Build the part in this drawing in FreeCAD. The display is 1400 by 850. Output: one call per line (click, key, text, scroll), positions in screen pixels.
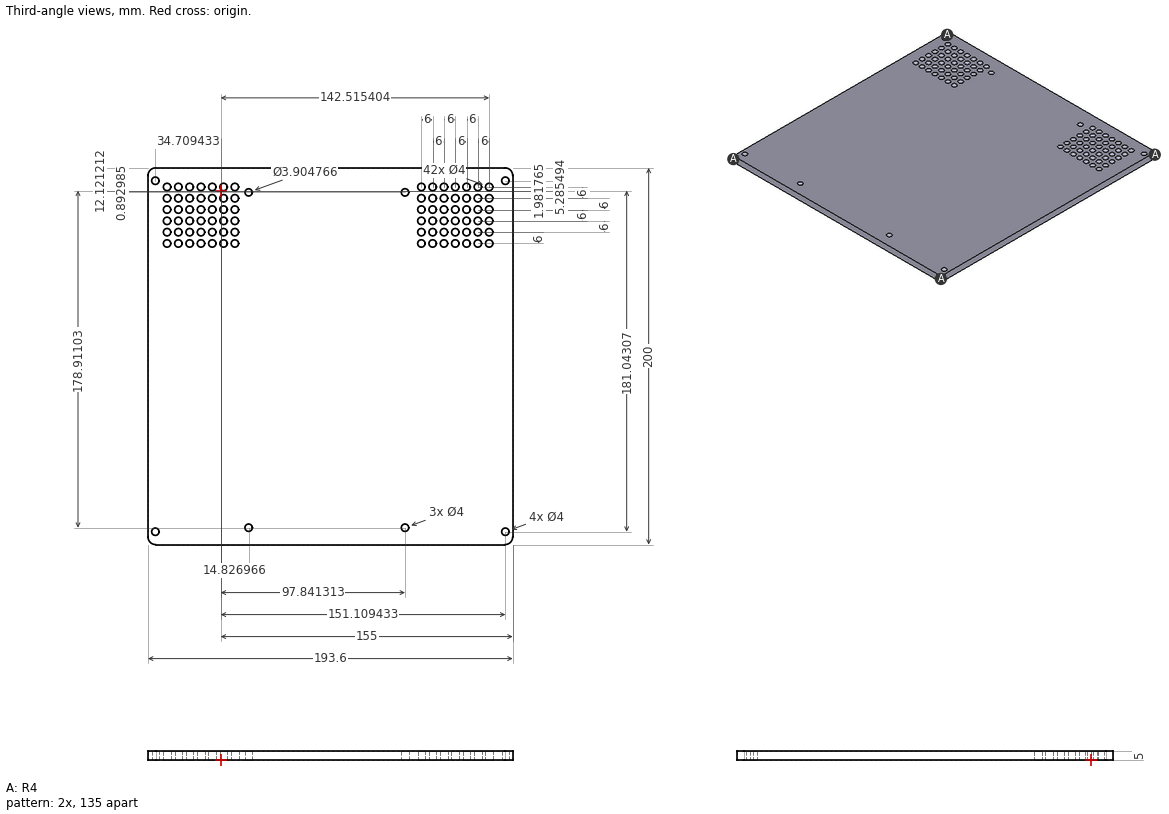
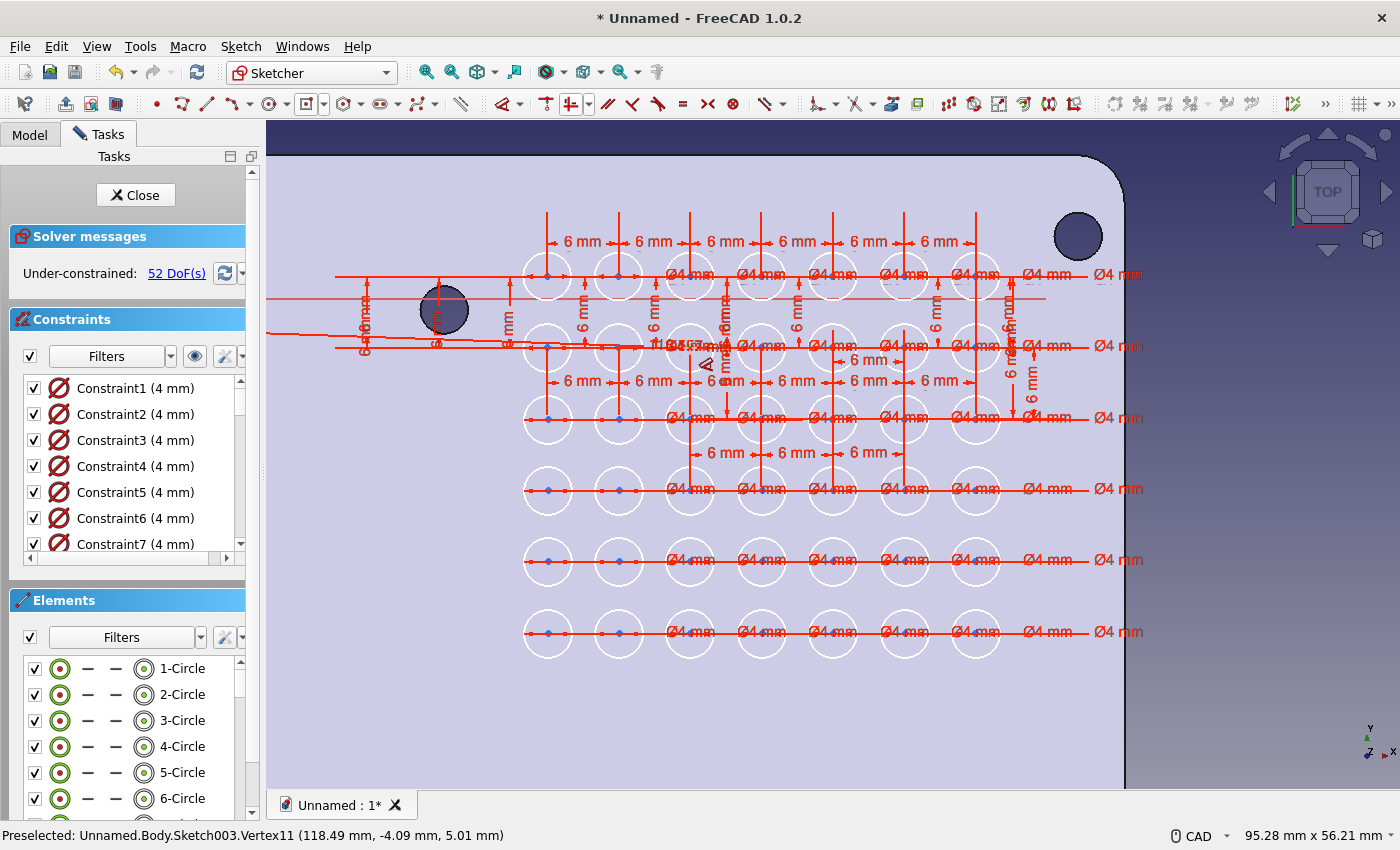
click(690, 420)
click(510, 384)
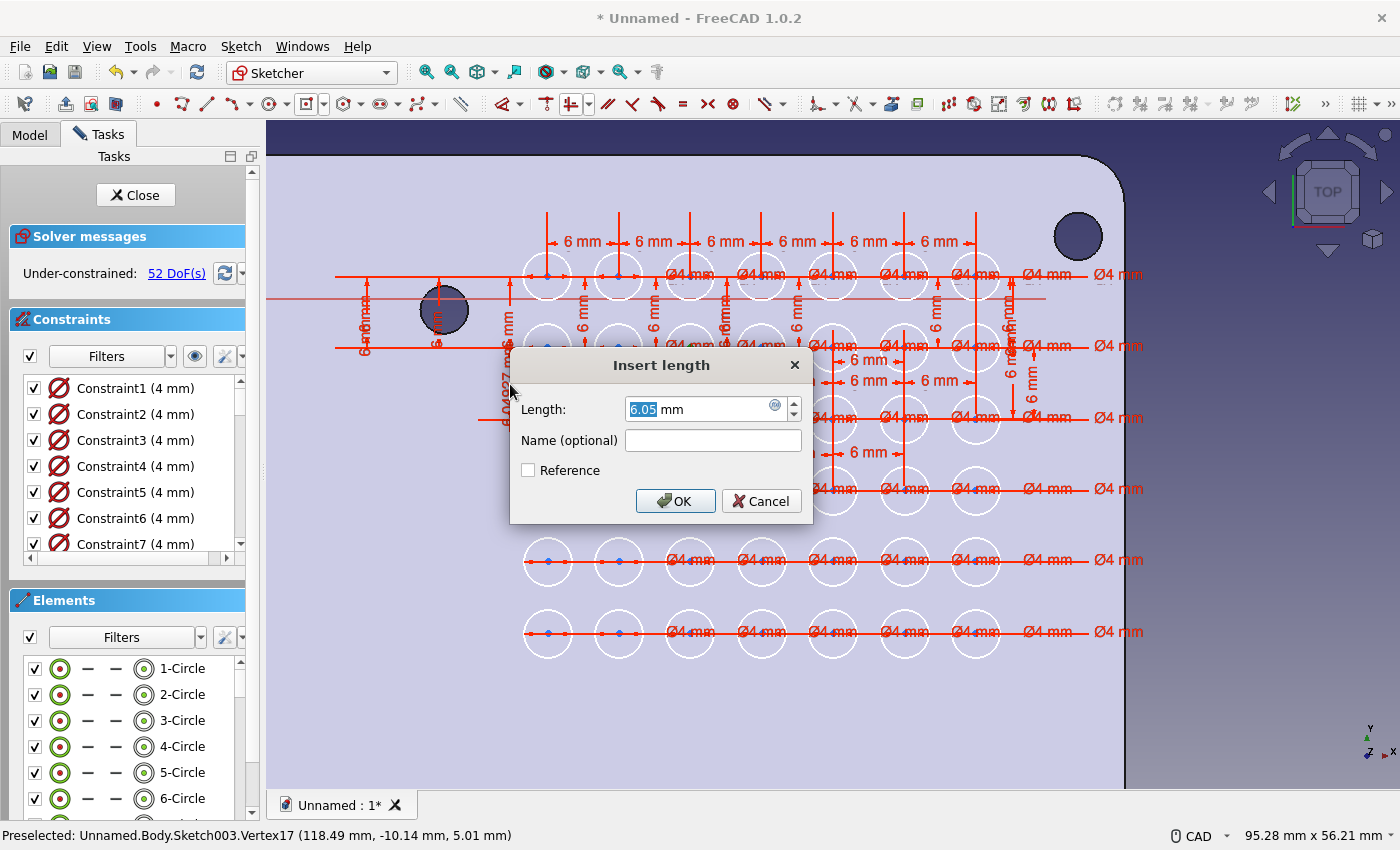
text(6)
key(Return)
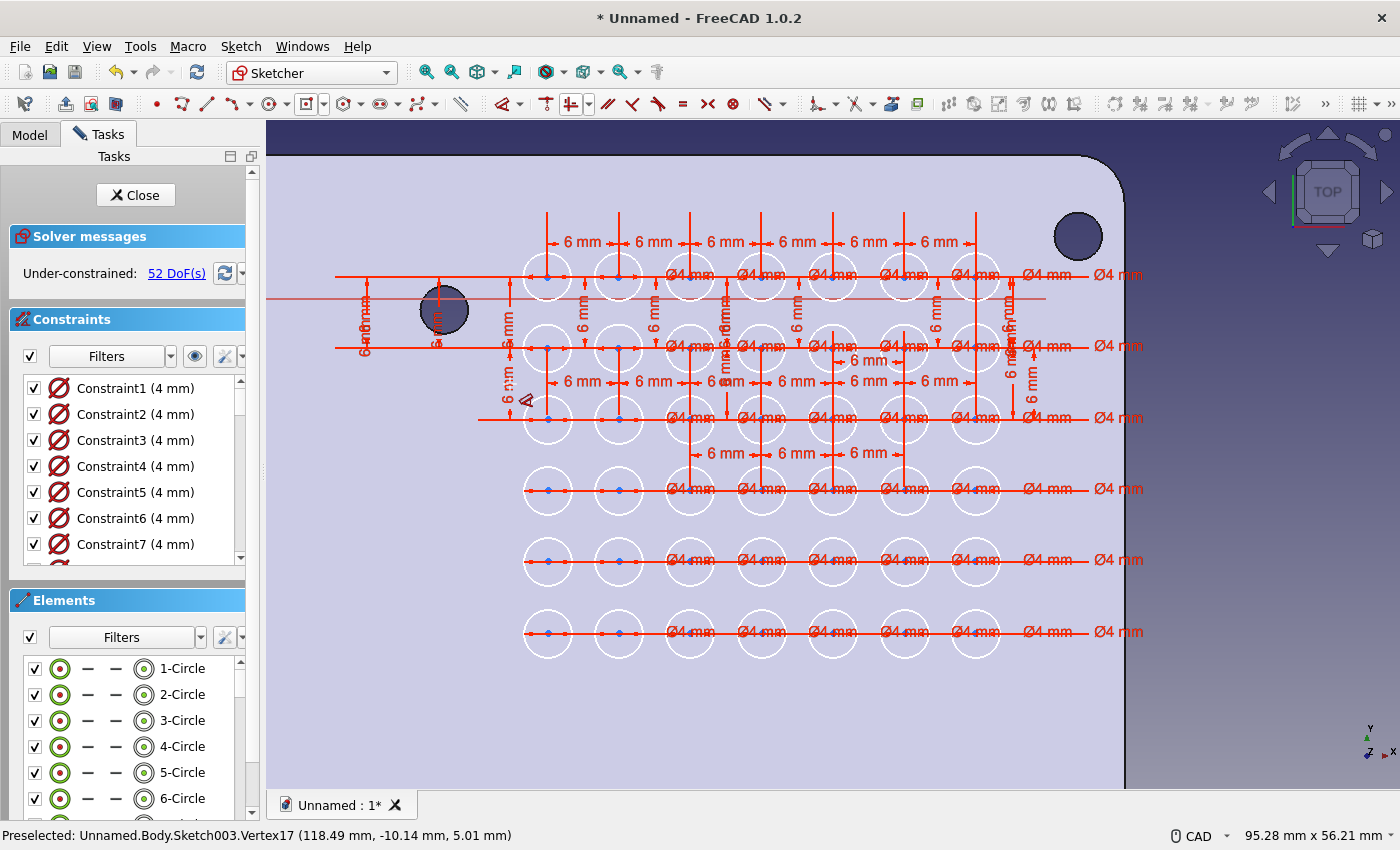
click(690, 420)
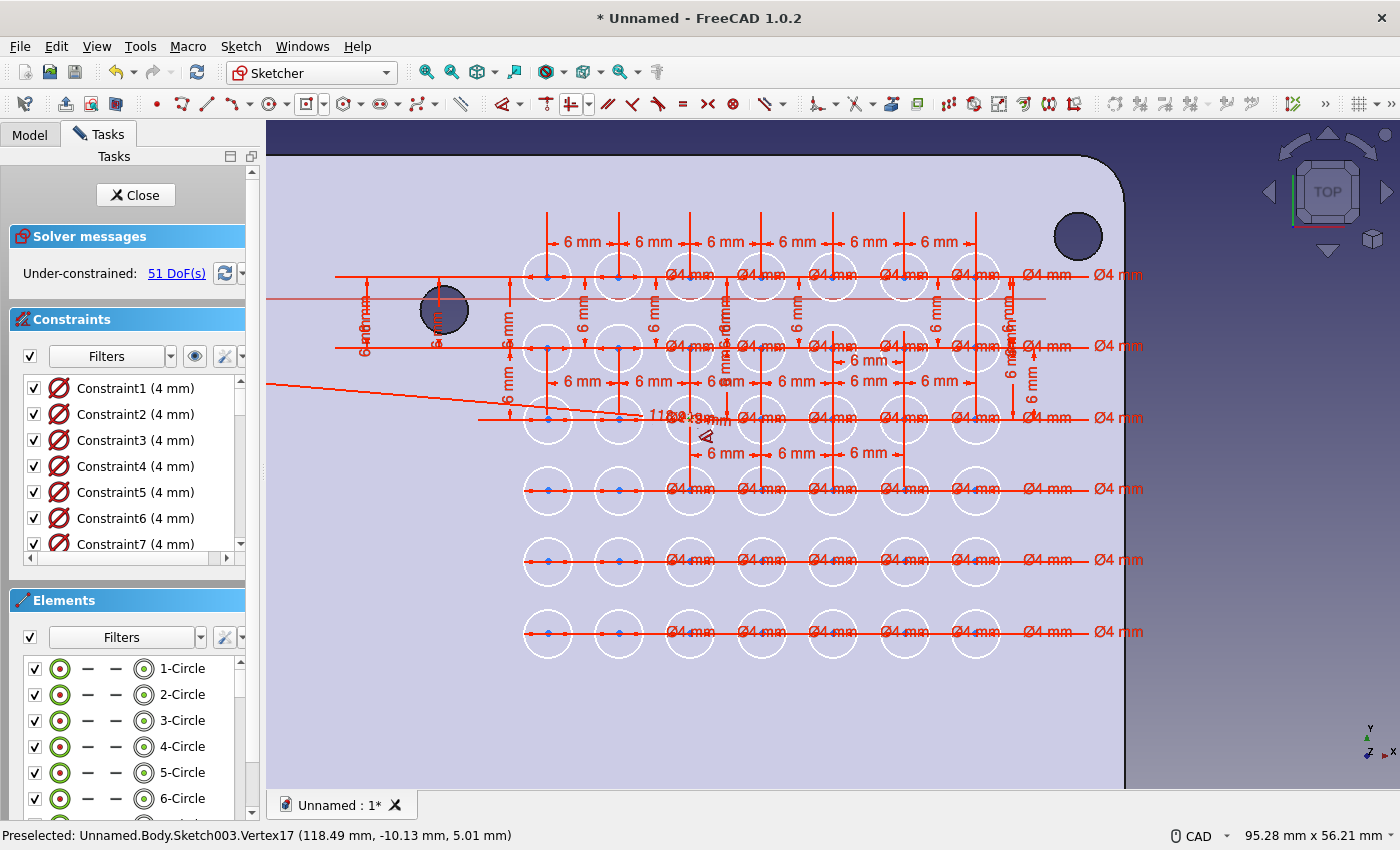
click(619, 420)
click(654, 454)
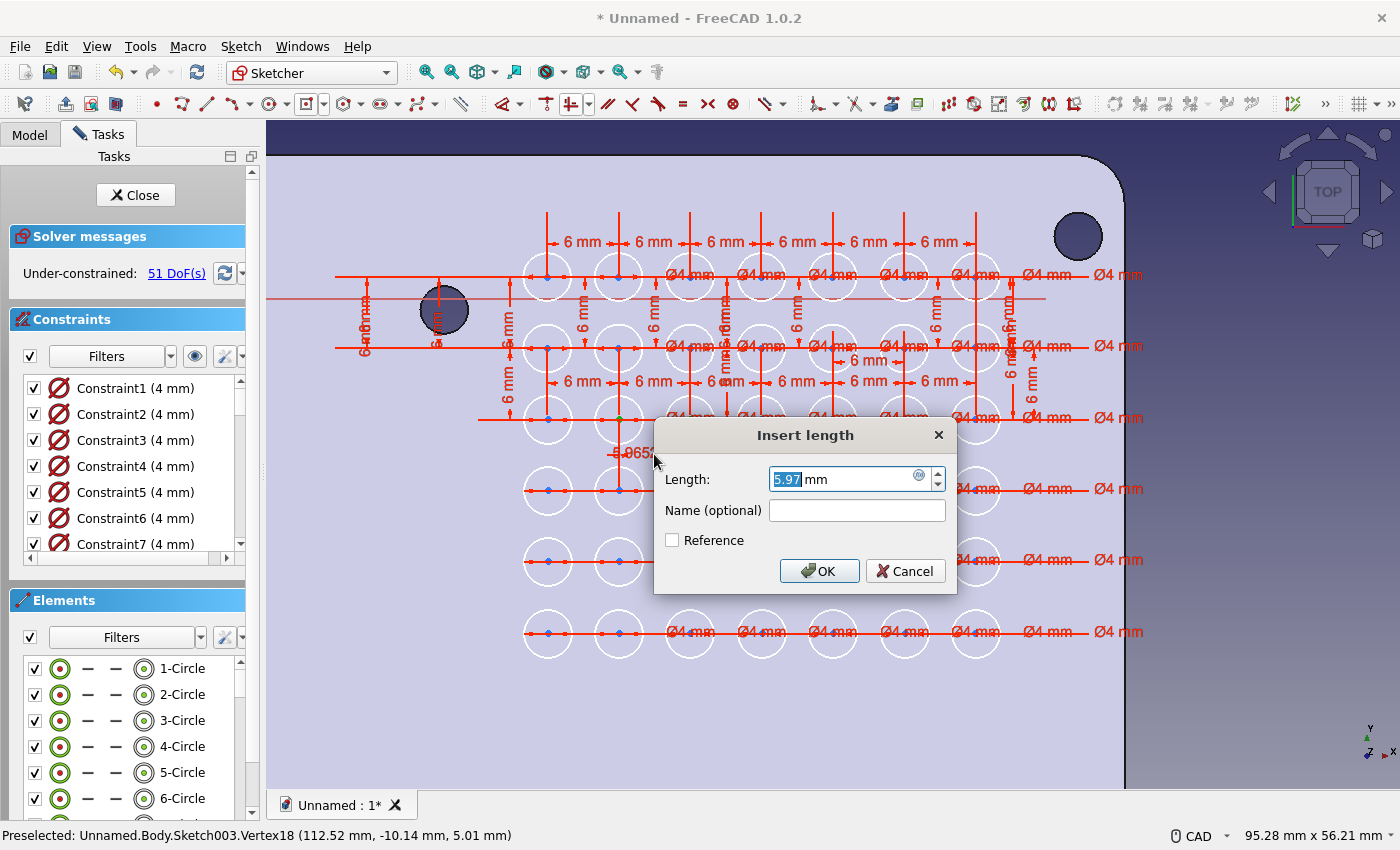
text(6)
key(Return)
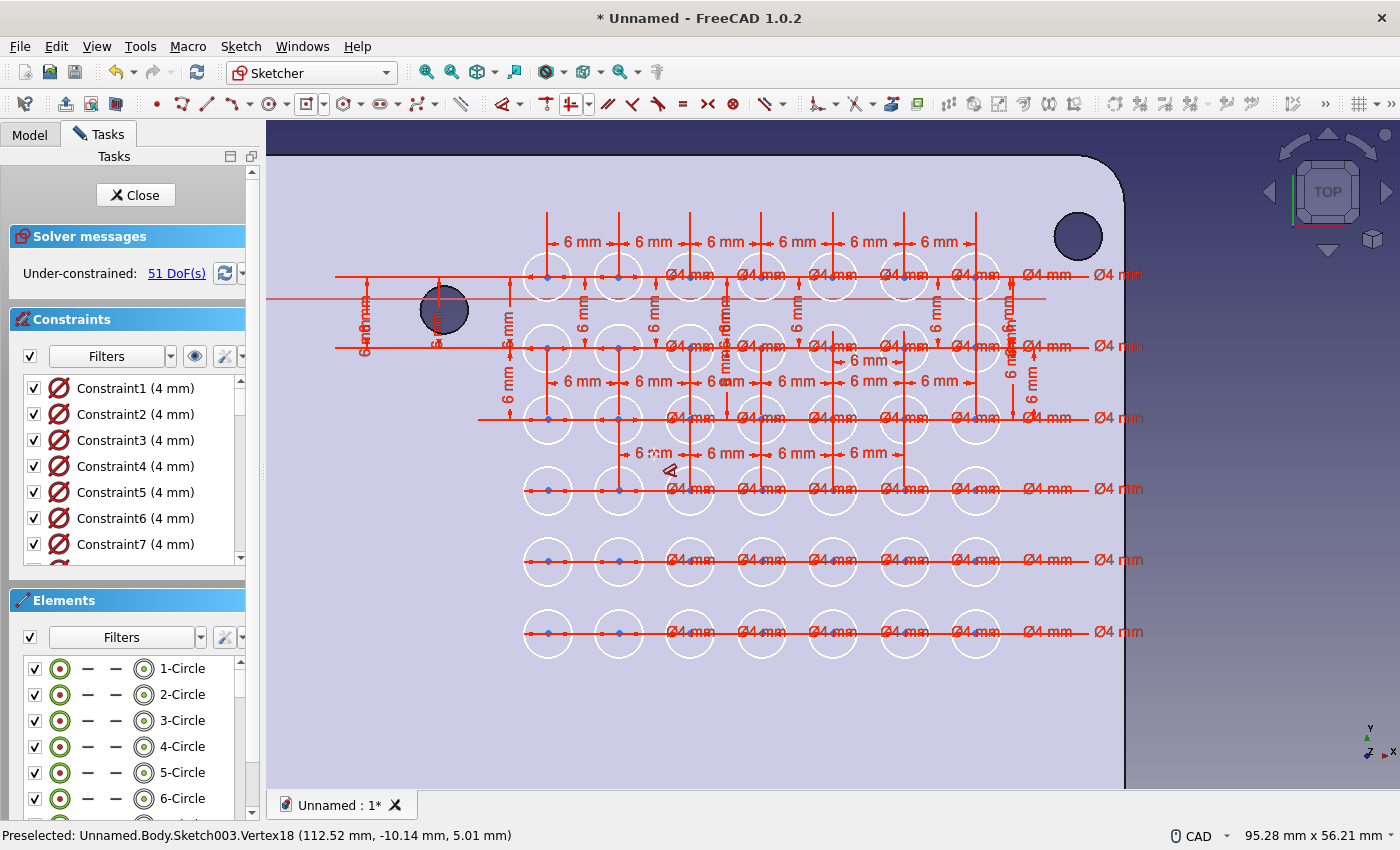
click(619, 348)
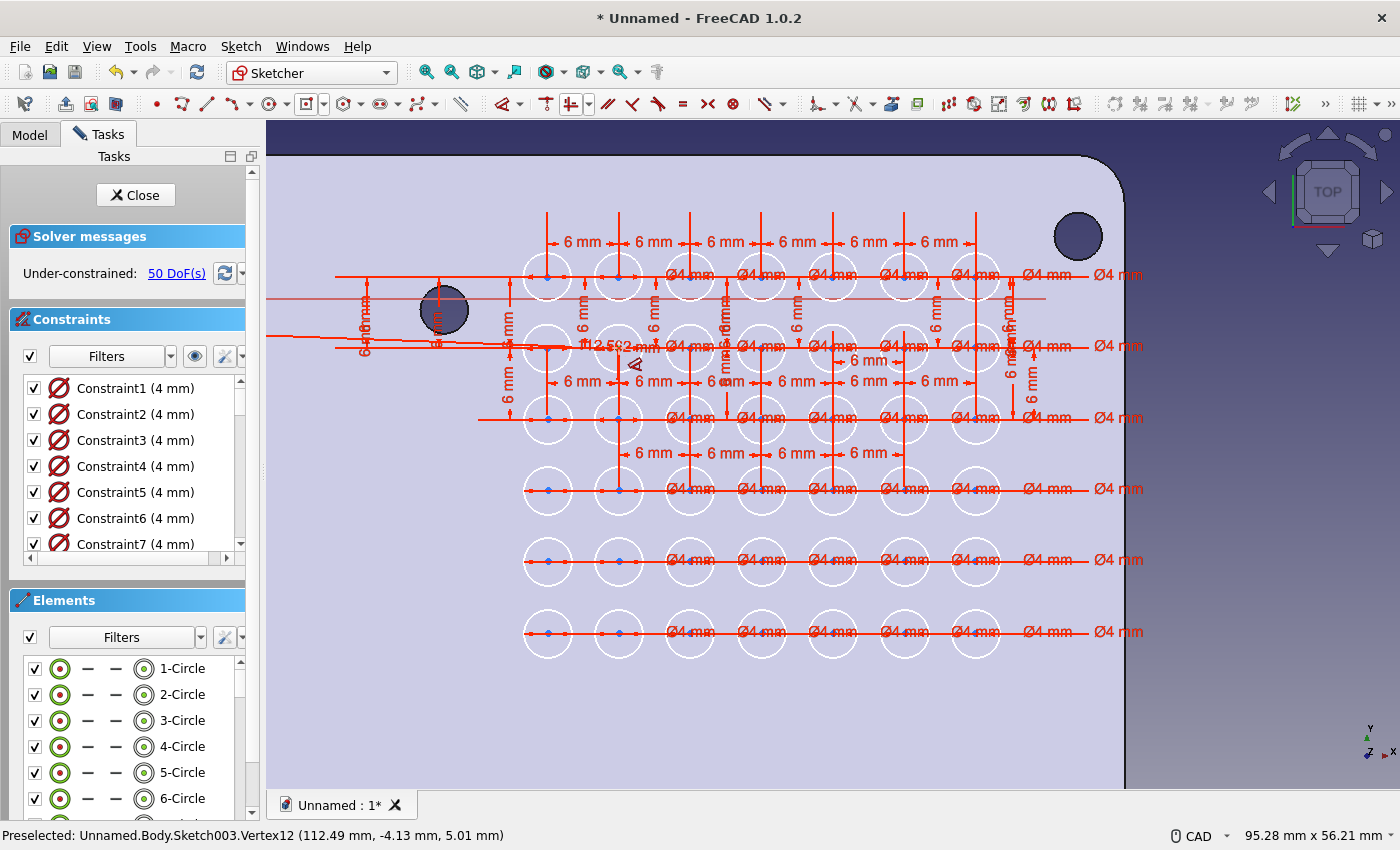
click(619, 420)
click(513, 409)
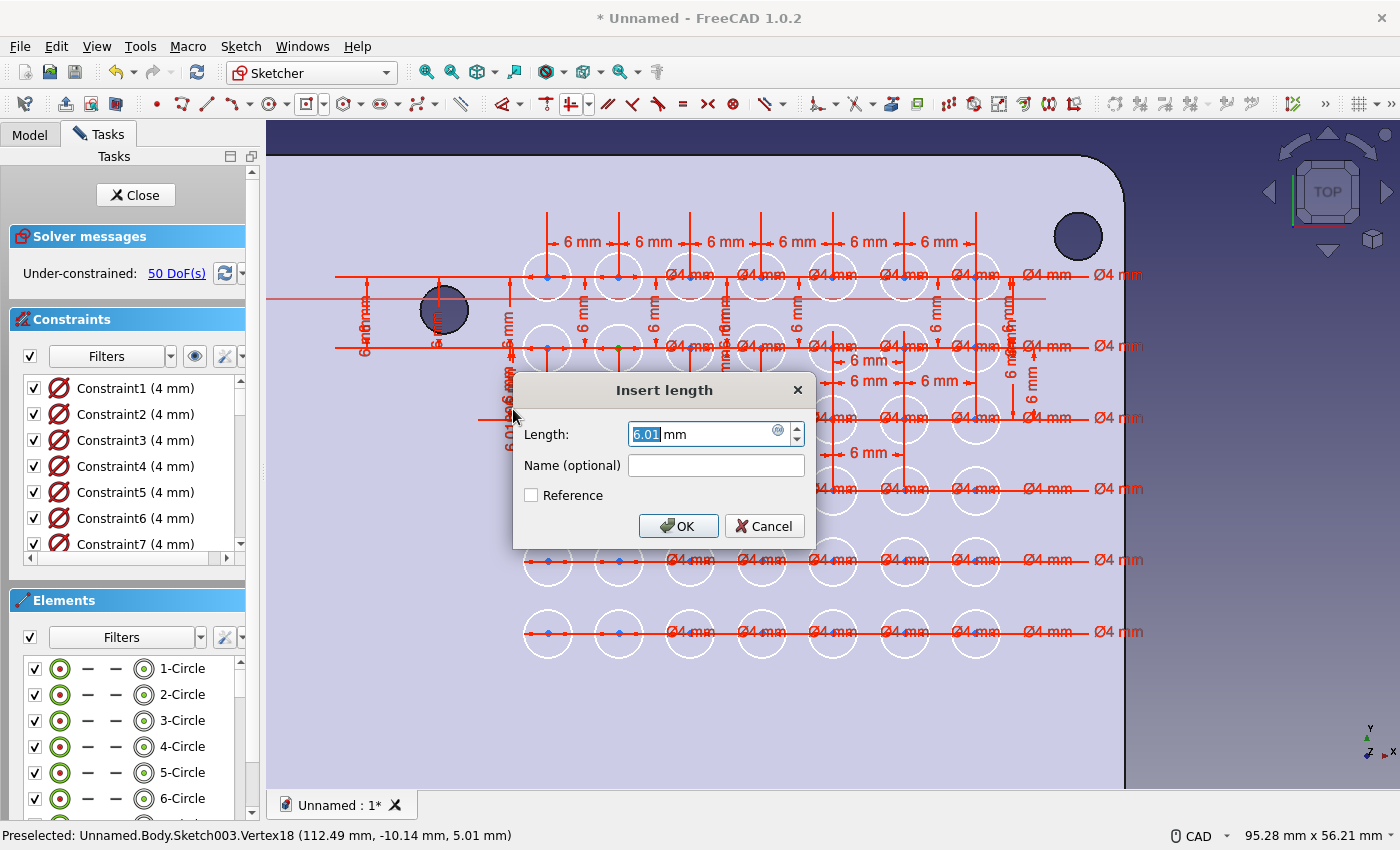
text(6)
key(Return)